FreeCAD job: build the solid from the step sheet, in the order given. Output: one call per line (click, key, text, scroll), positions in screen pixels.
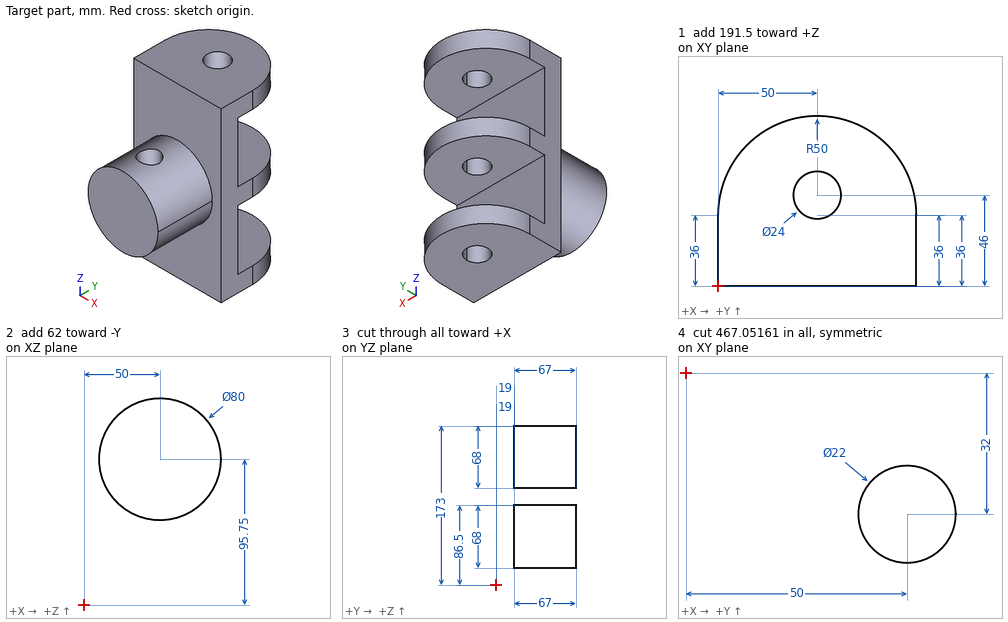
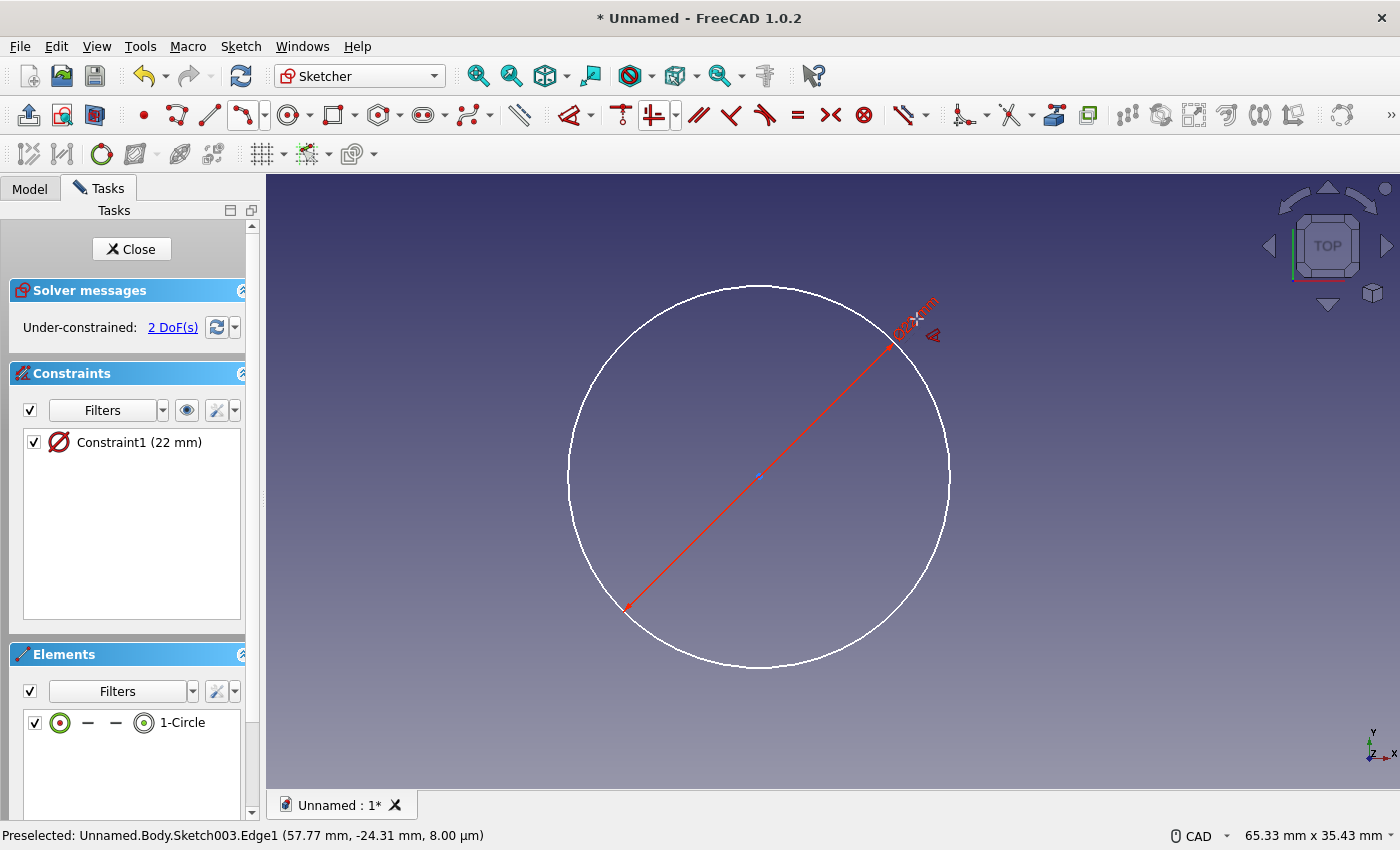
click(759, 477)
click(527, 511)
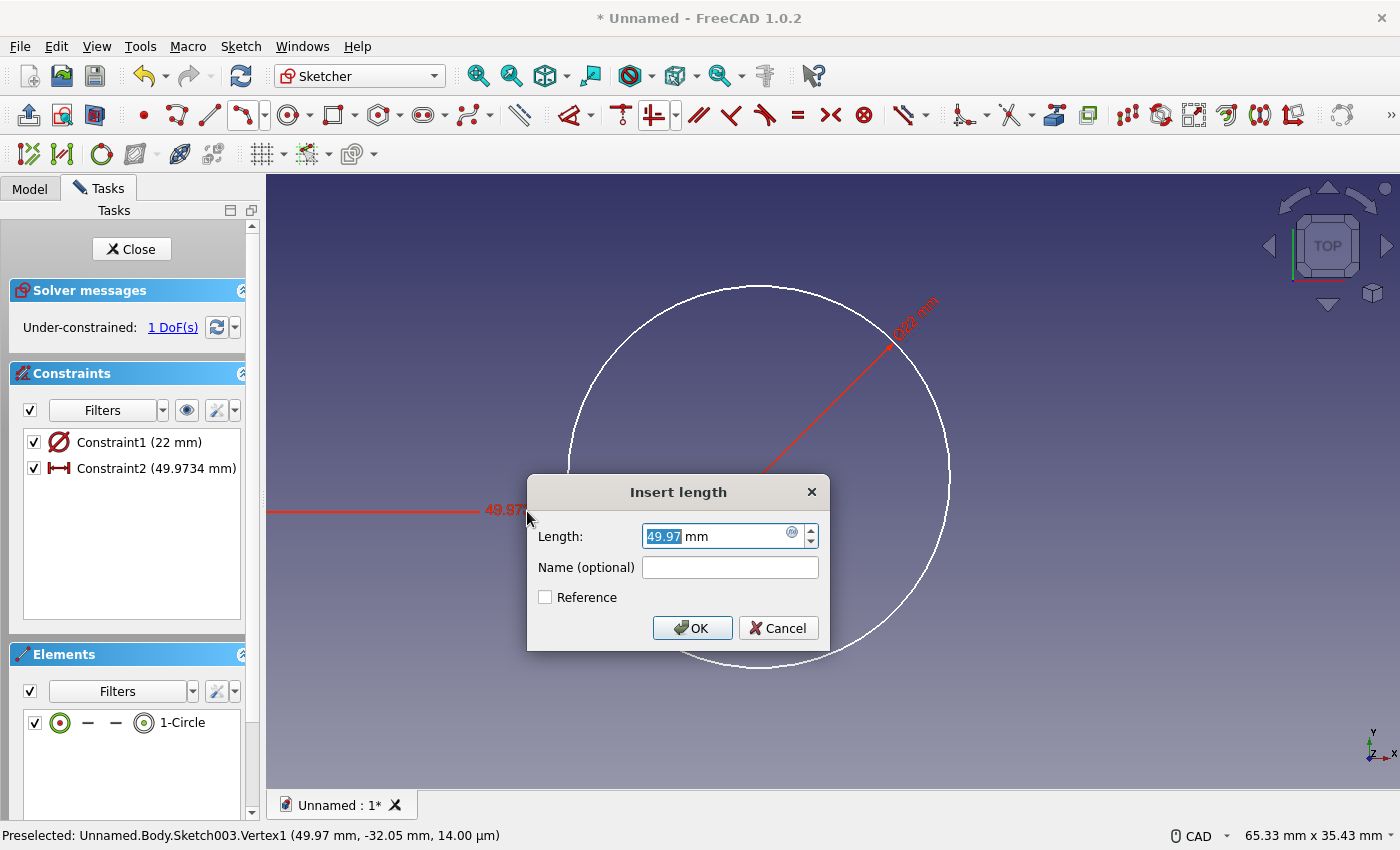
text(50)
key(Return)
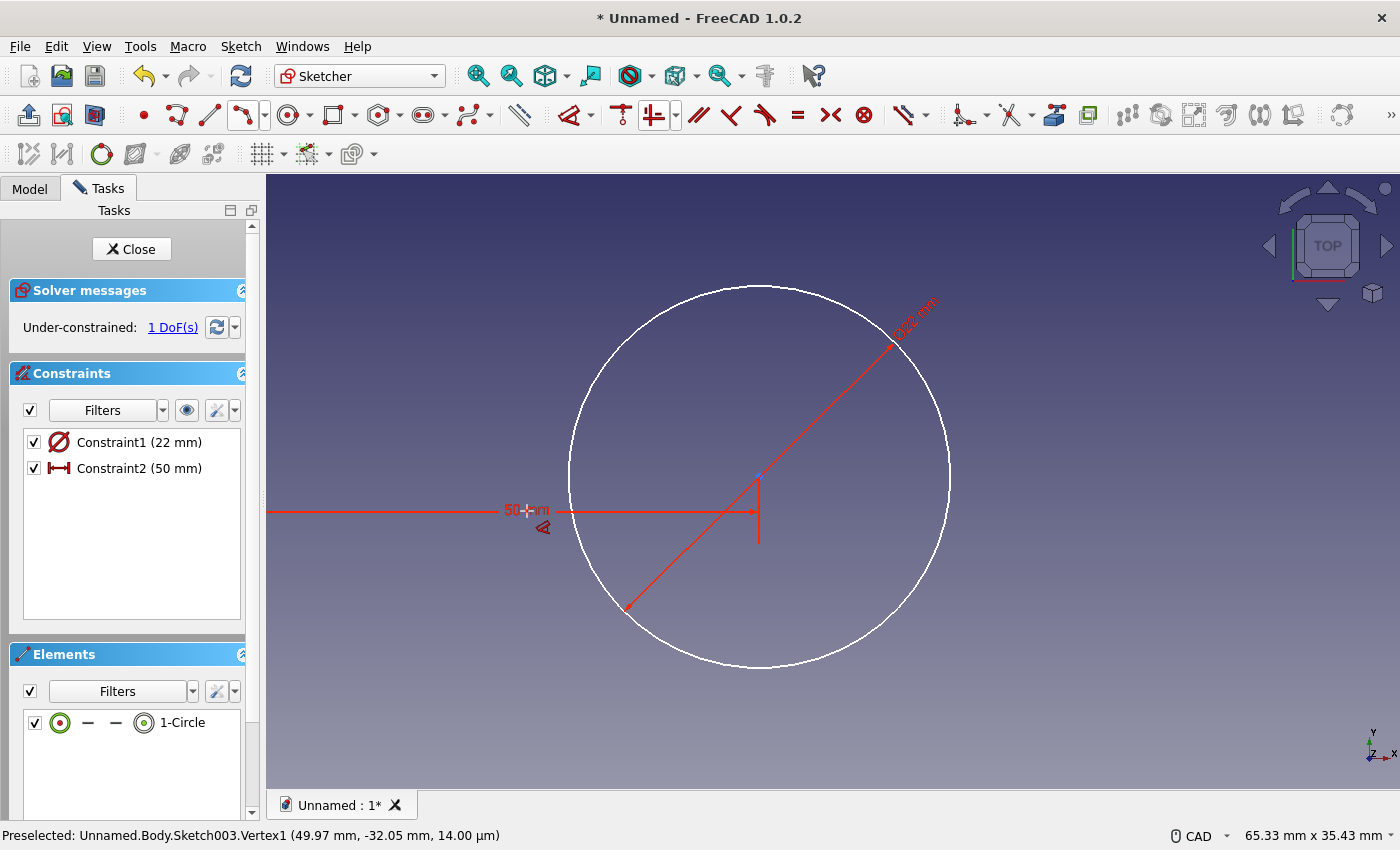
click(759, 477)
click(793, 339)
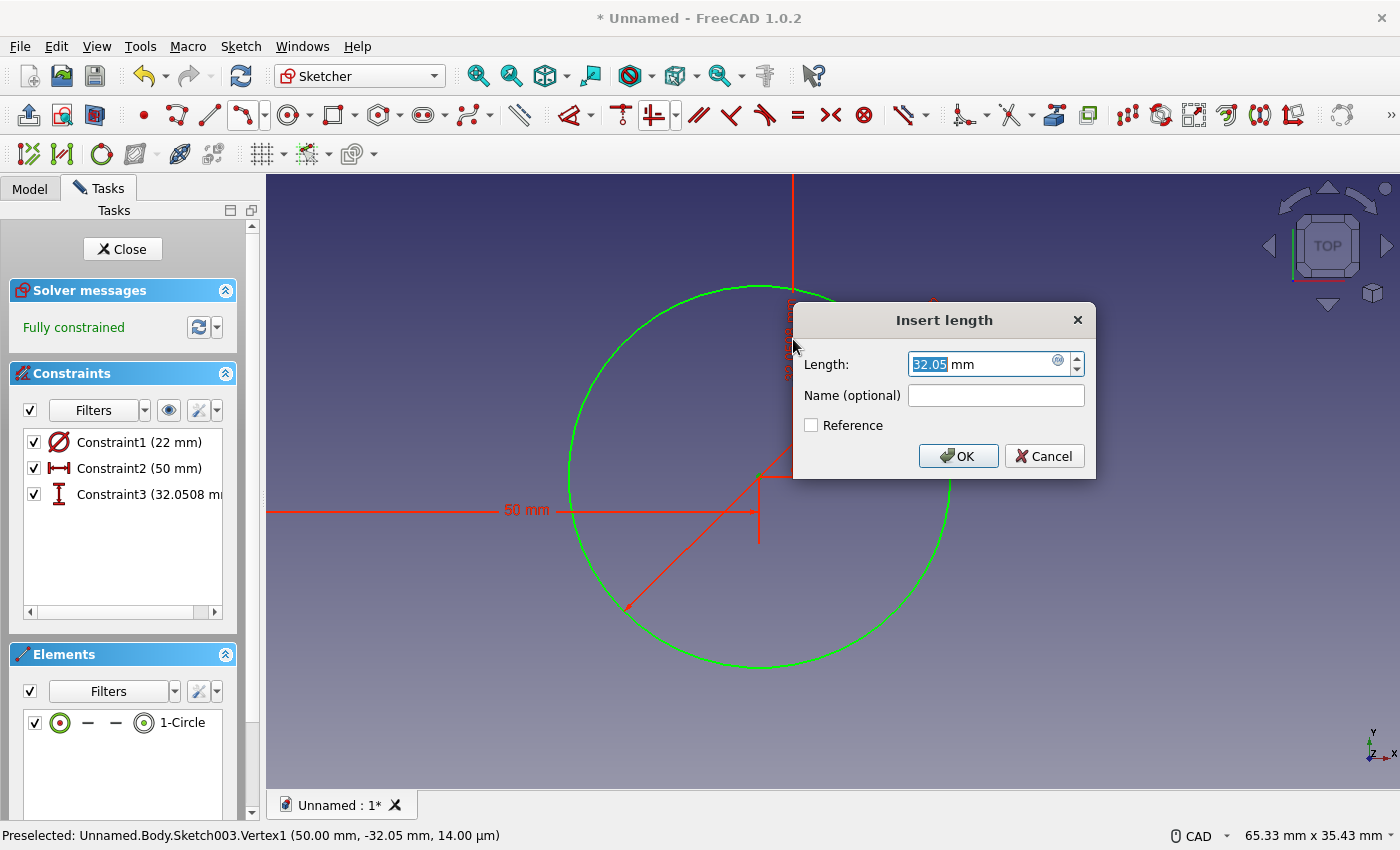
text(32)
key(Return)
key(Escape)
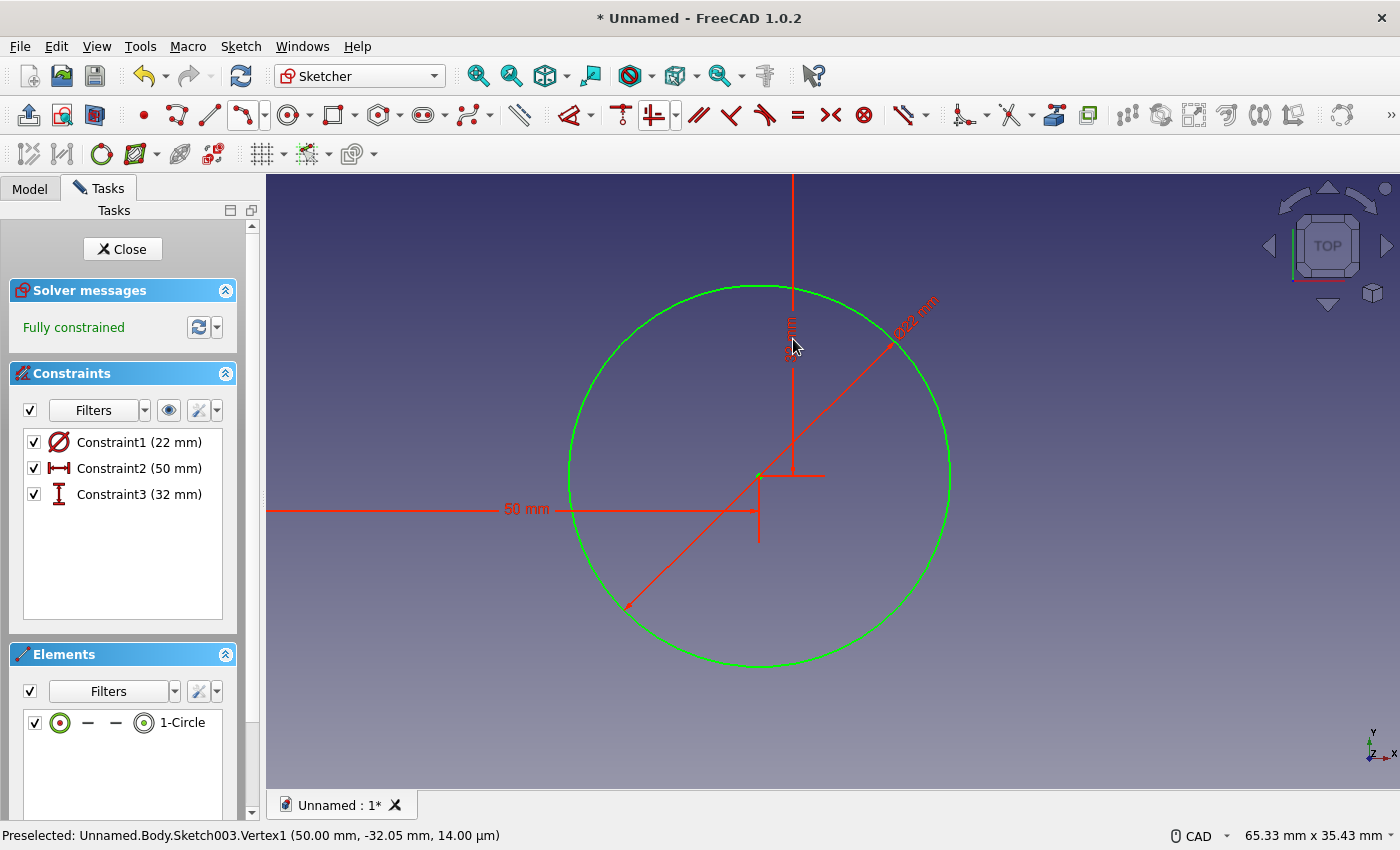
click(123, 249)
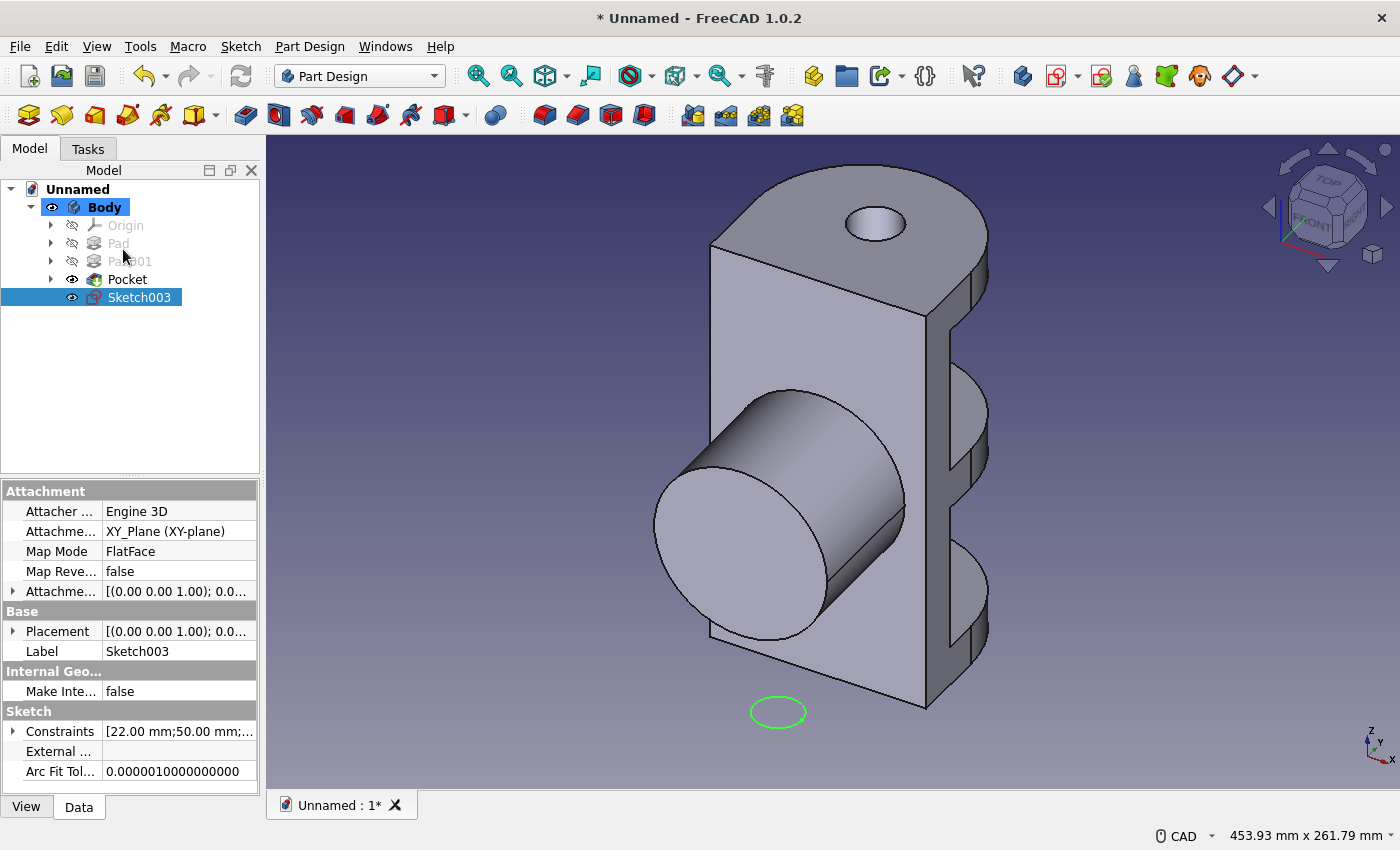
click(246, 116)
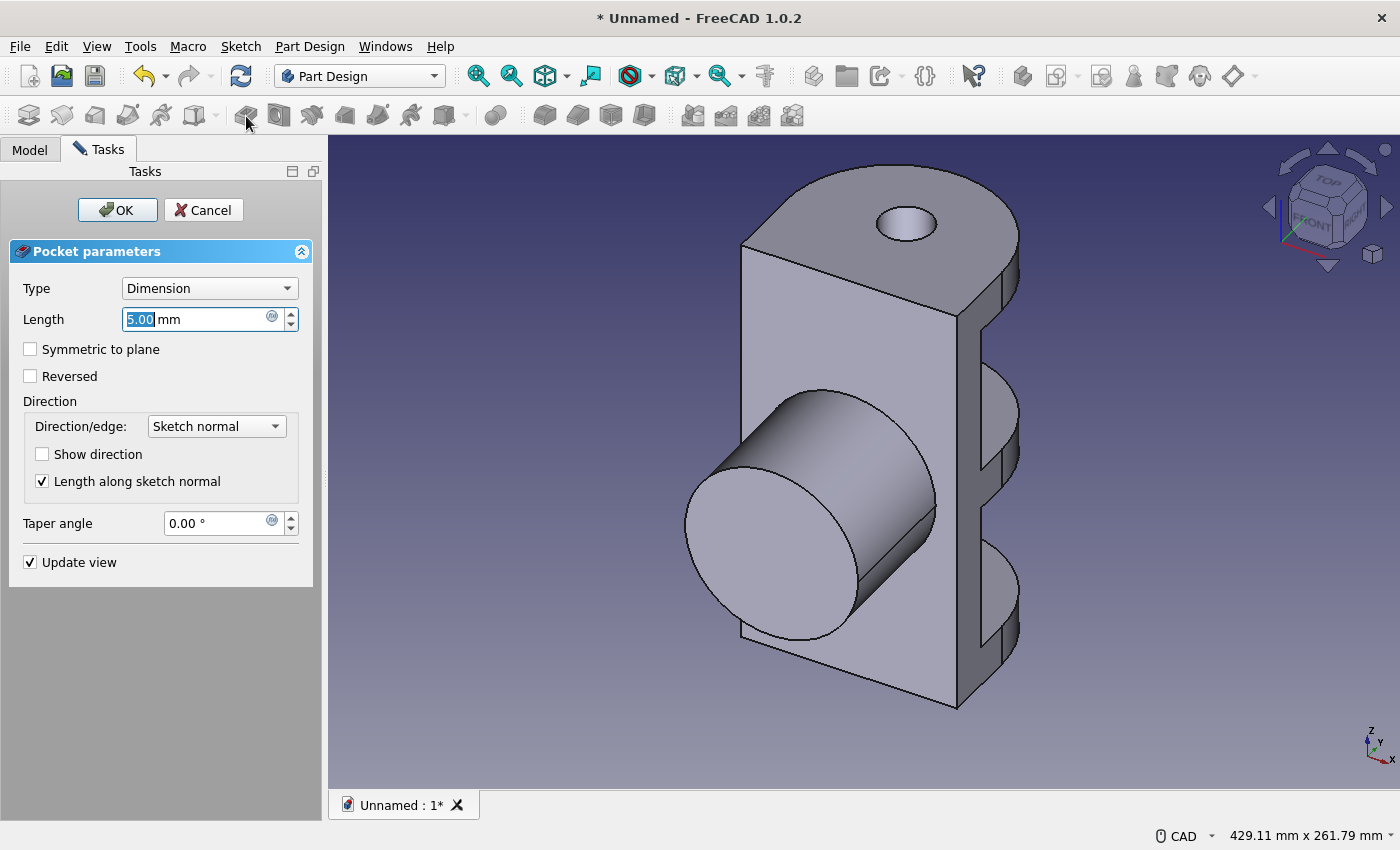
text(467.05161)
key(Tab)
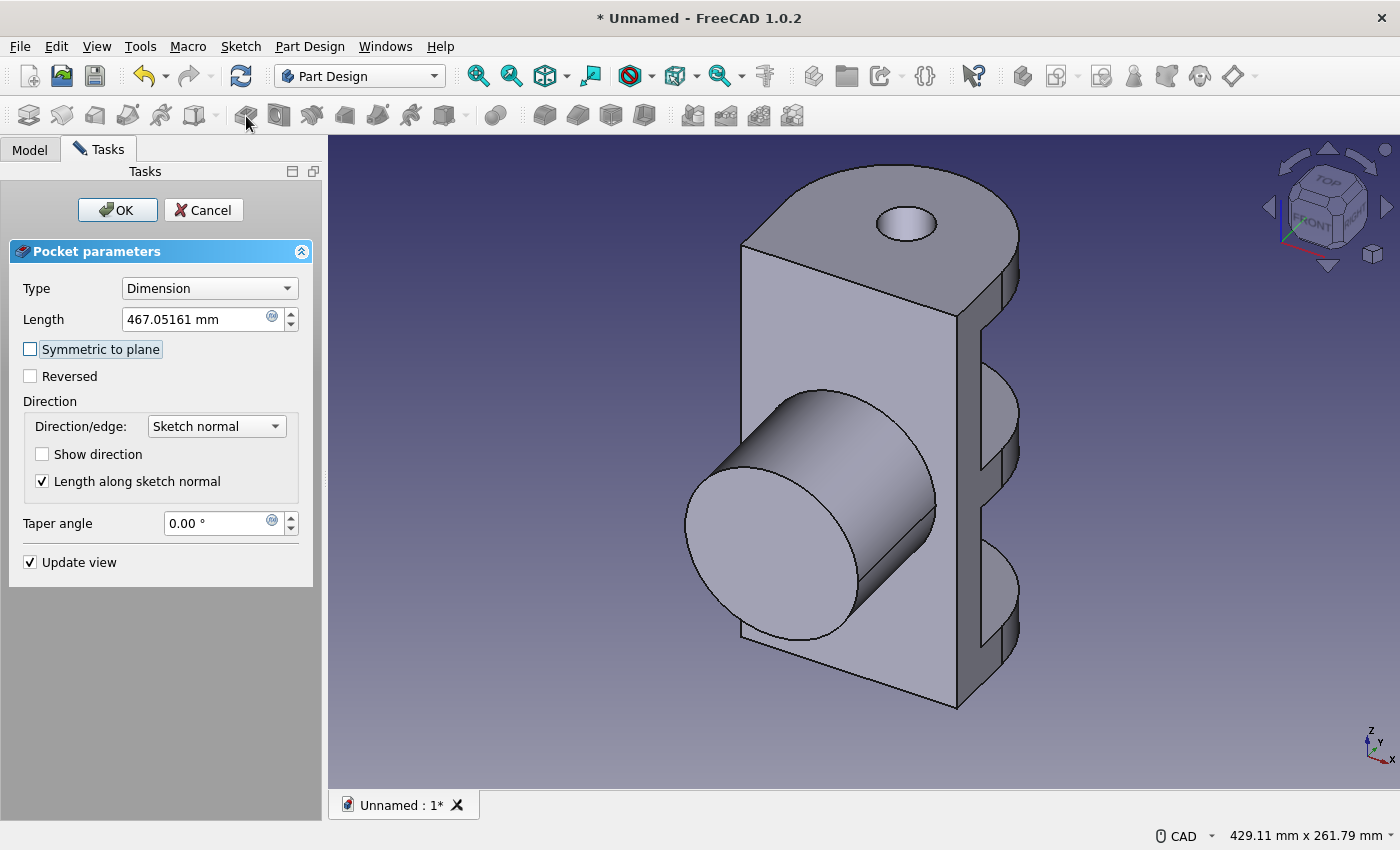
click(31, 349)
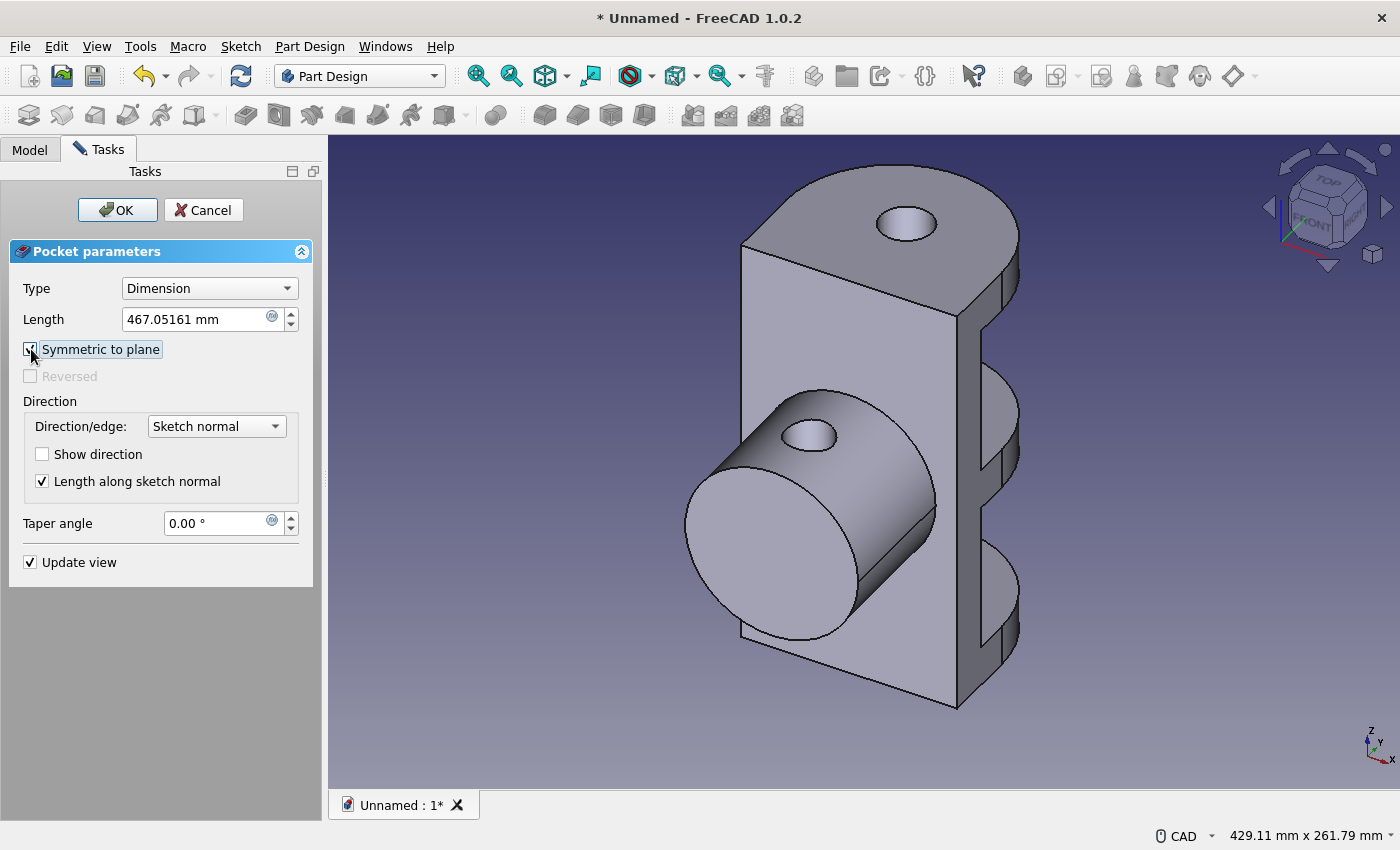
click(118, 210)